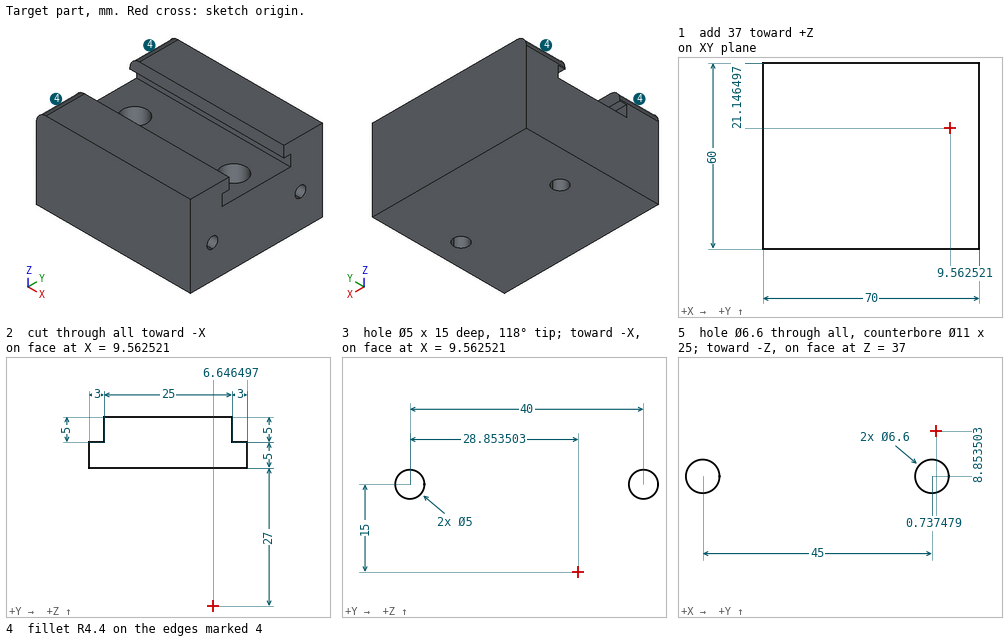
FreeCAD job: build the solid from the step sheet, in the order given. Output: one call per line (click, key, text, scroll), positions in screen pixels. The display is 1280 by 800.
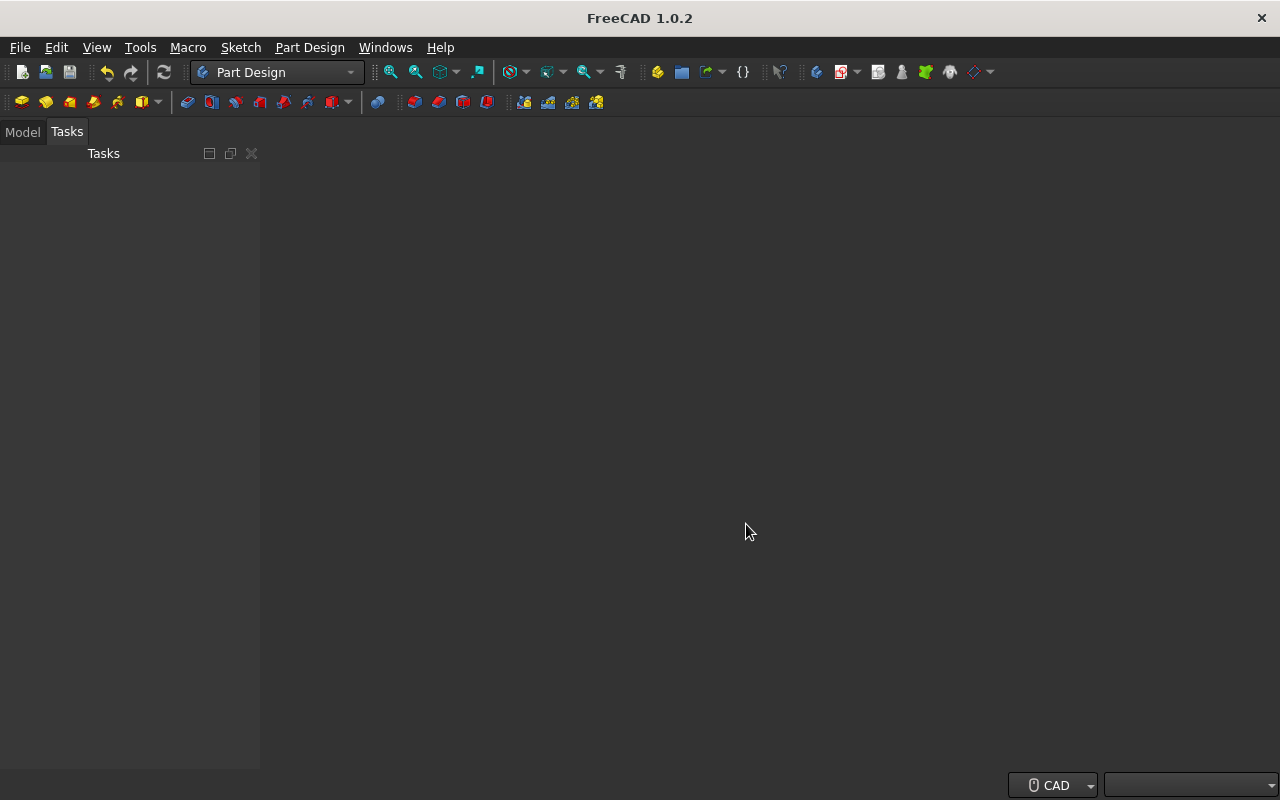
click(22, 72)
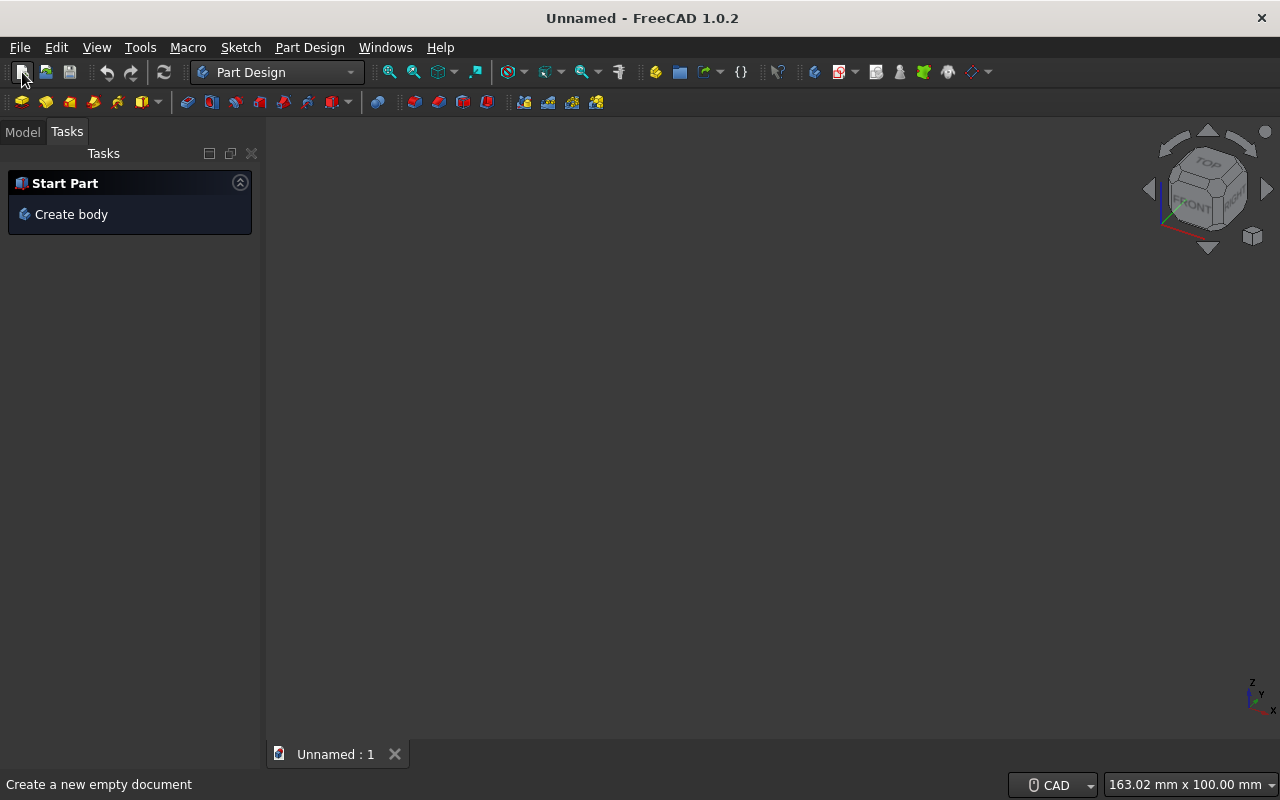
click(840, 72)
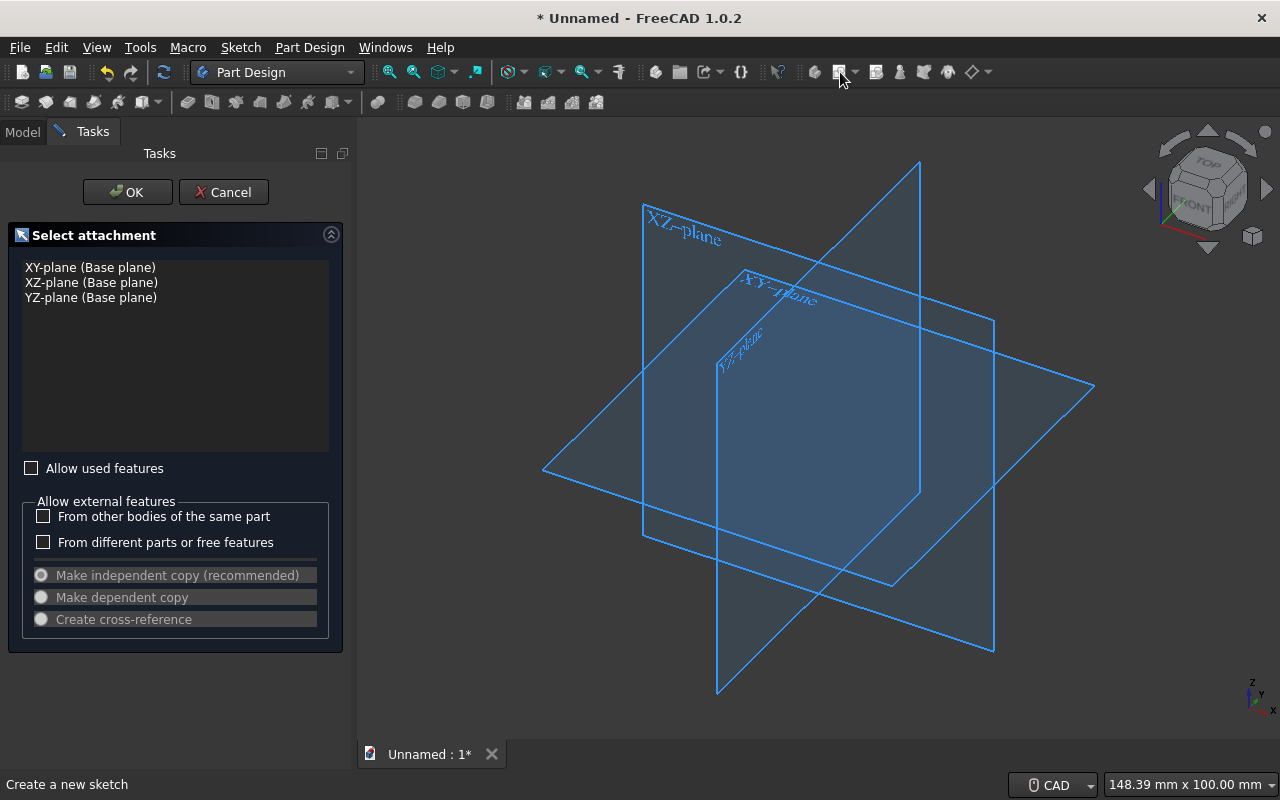
click(82, 268)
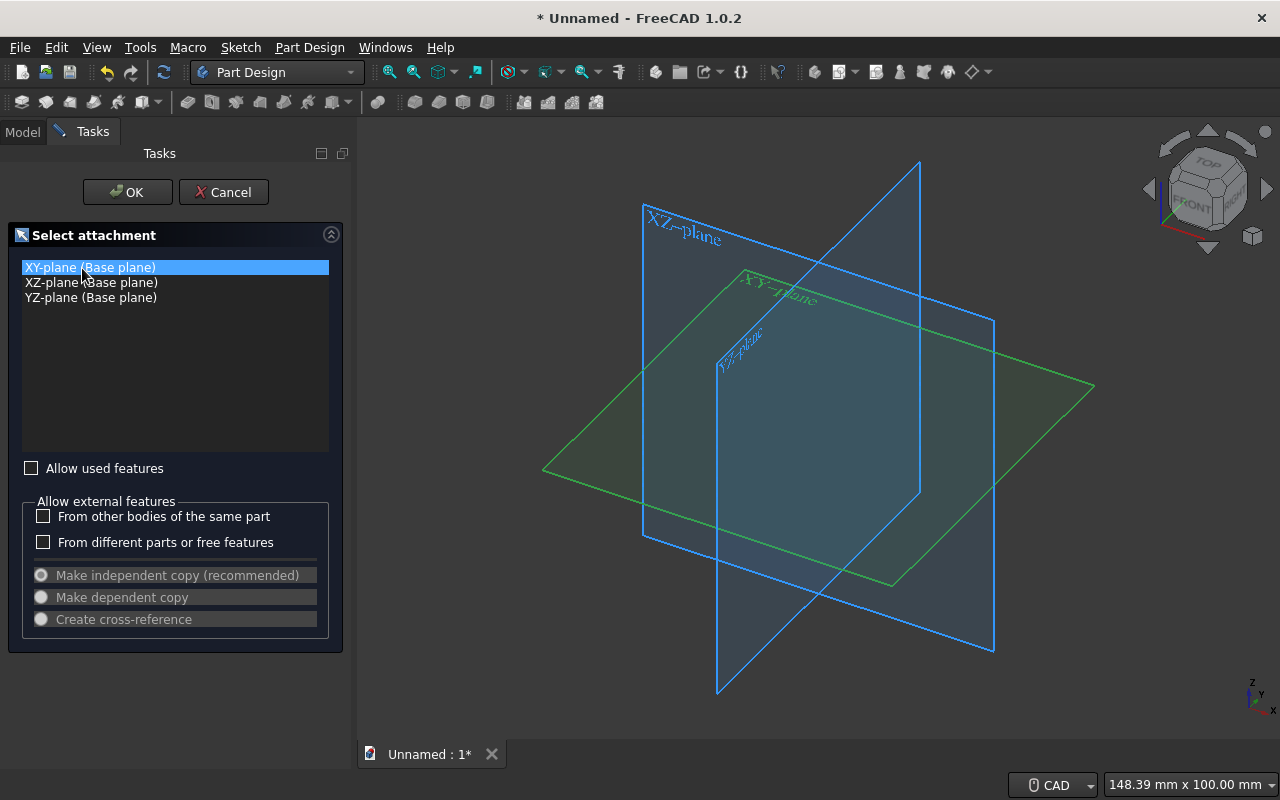
click(128, 192)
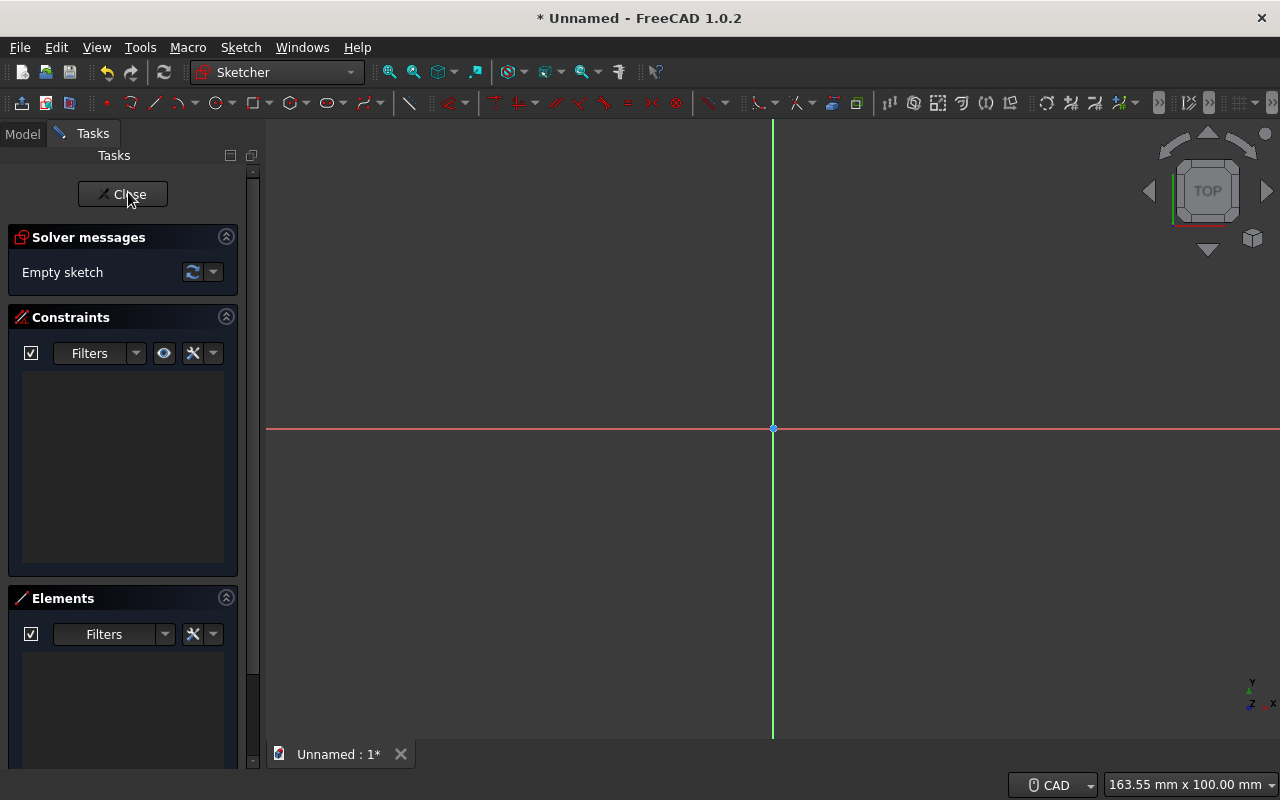
click(254, 104)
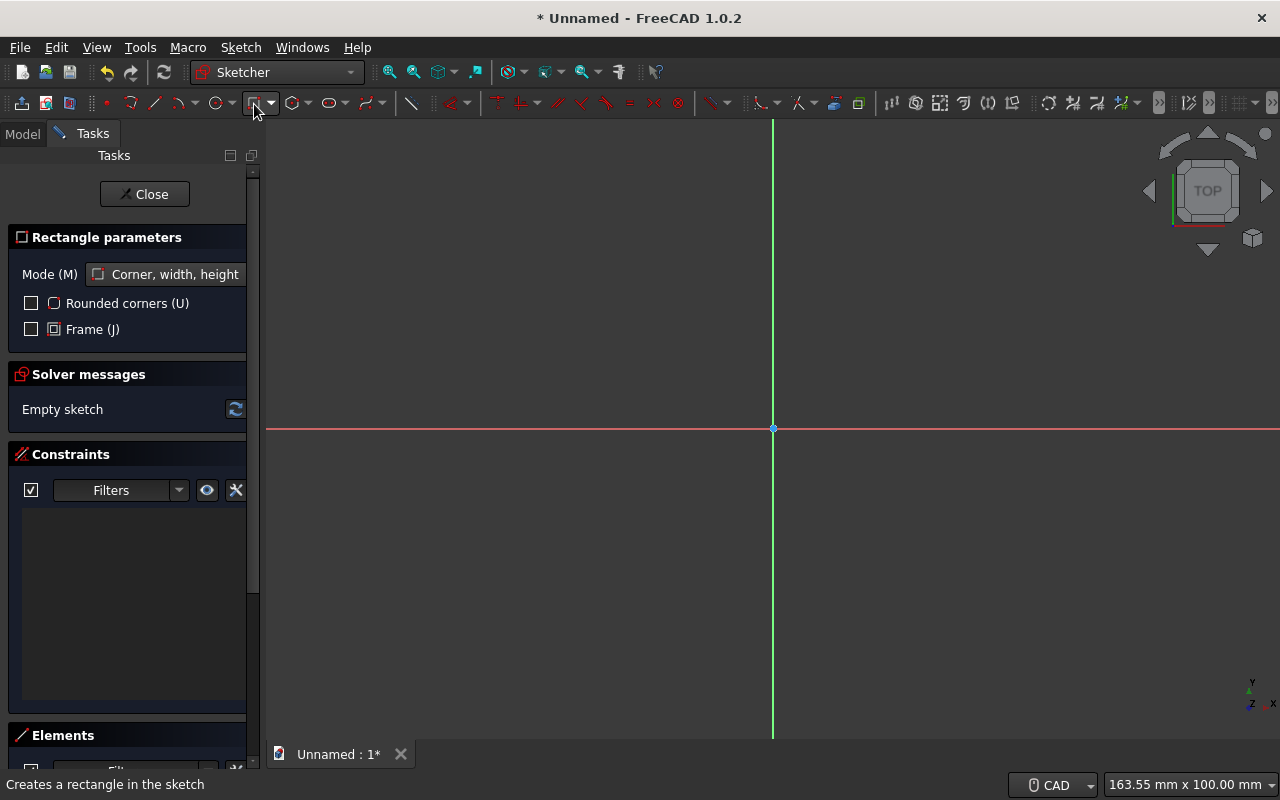
click(398, 298)
click(832, 670)
key(Escape)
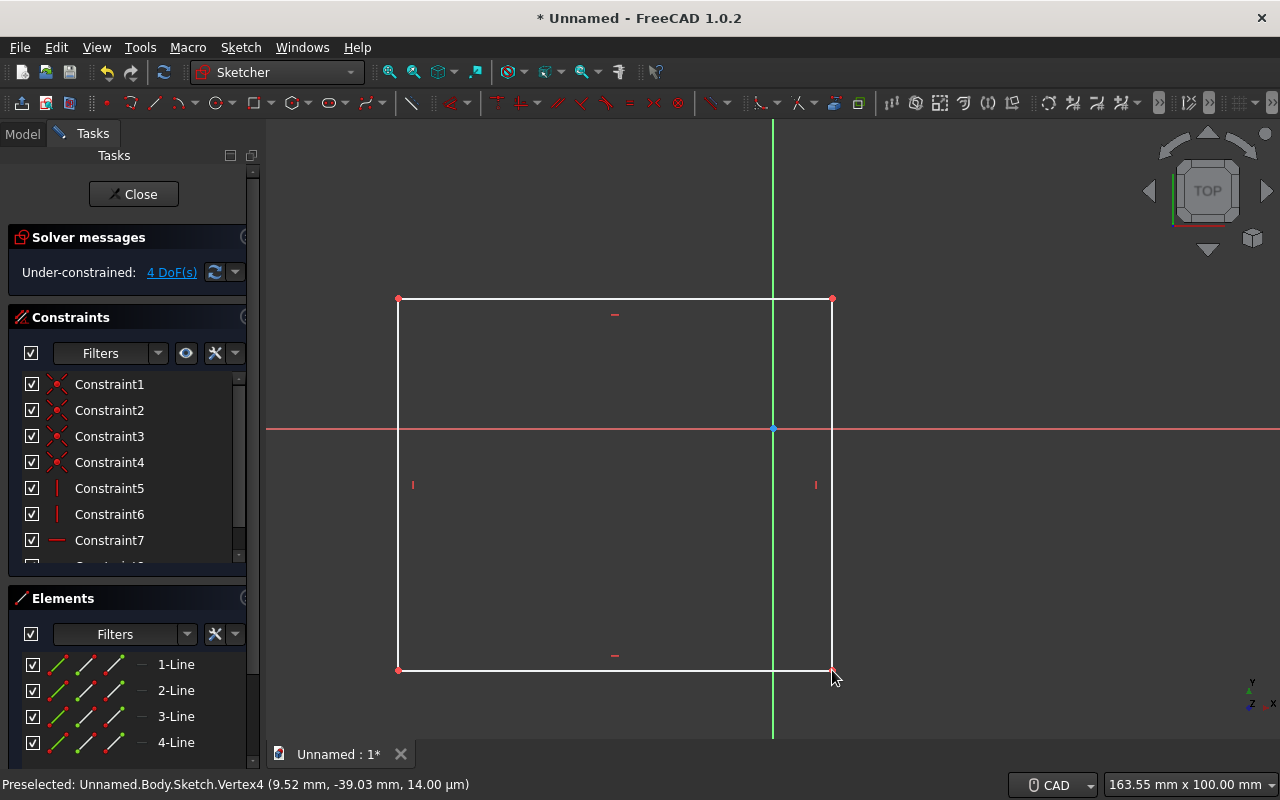
click(398, 411)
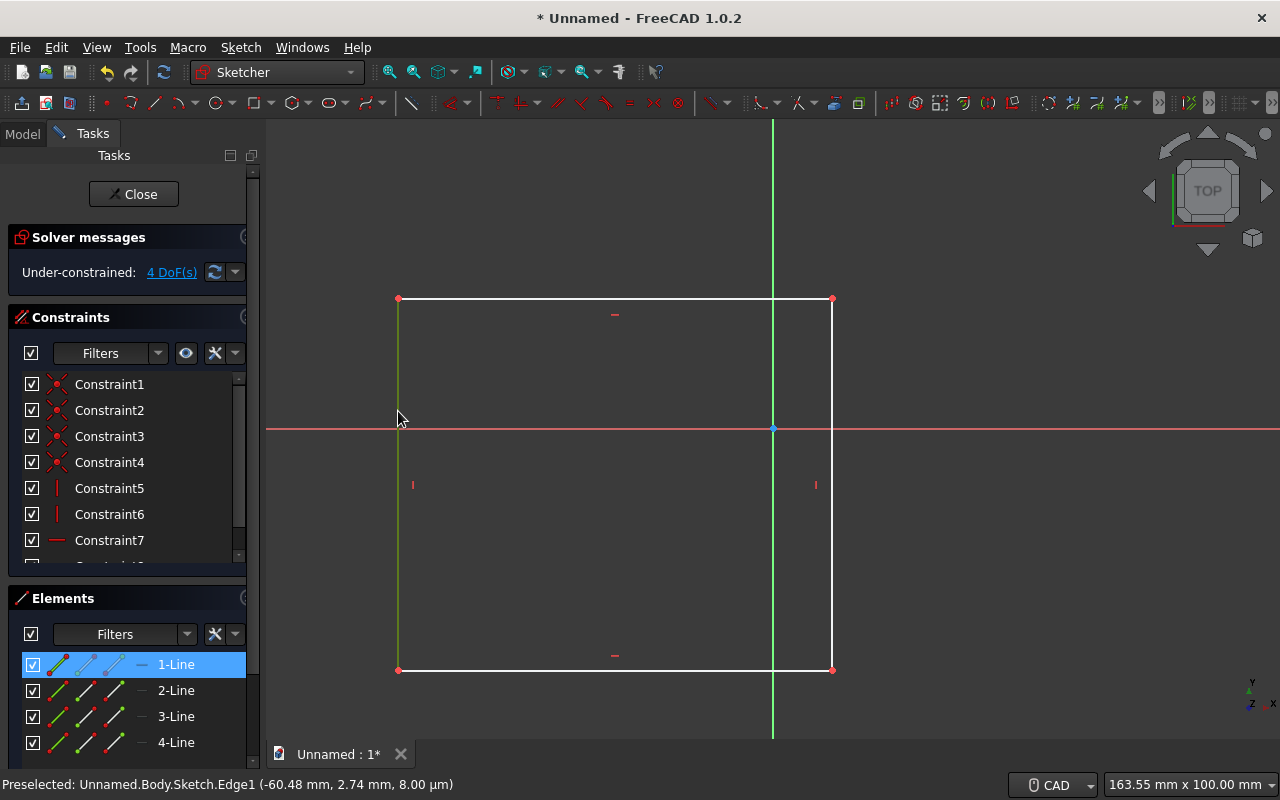
click(470, 104)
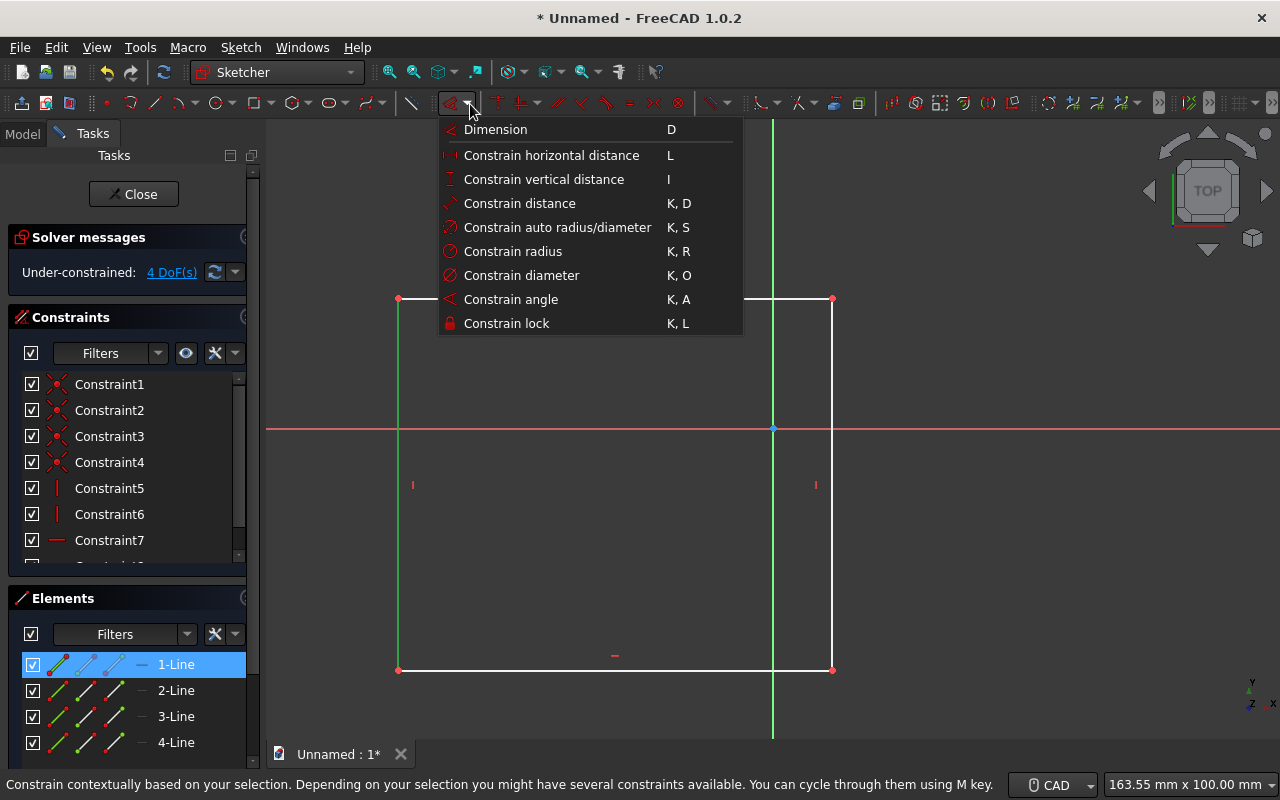
click(591, 179)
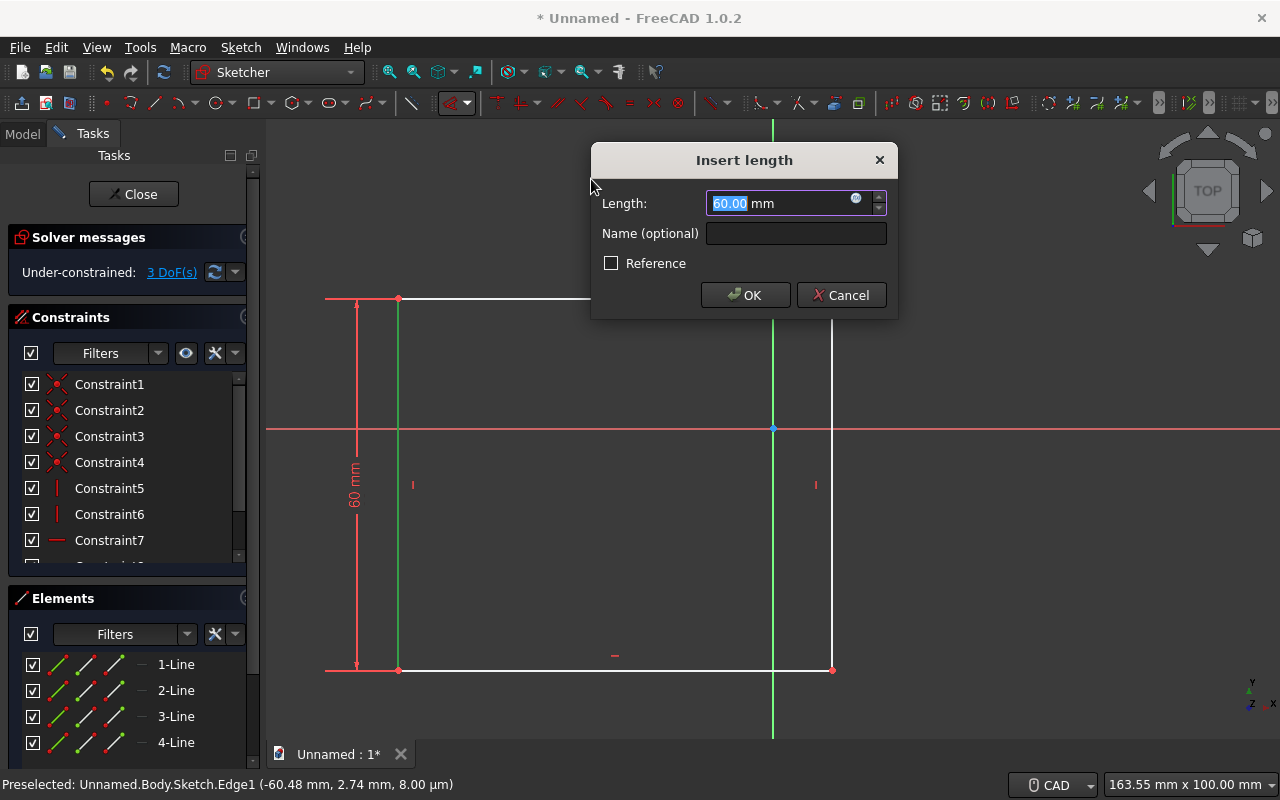
text(60)
key(Return)